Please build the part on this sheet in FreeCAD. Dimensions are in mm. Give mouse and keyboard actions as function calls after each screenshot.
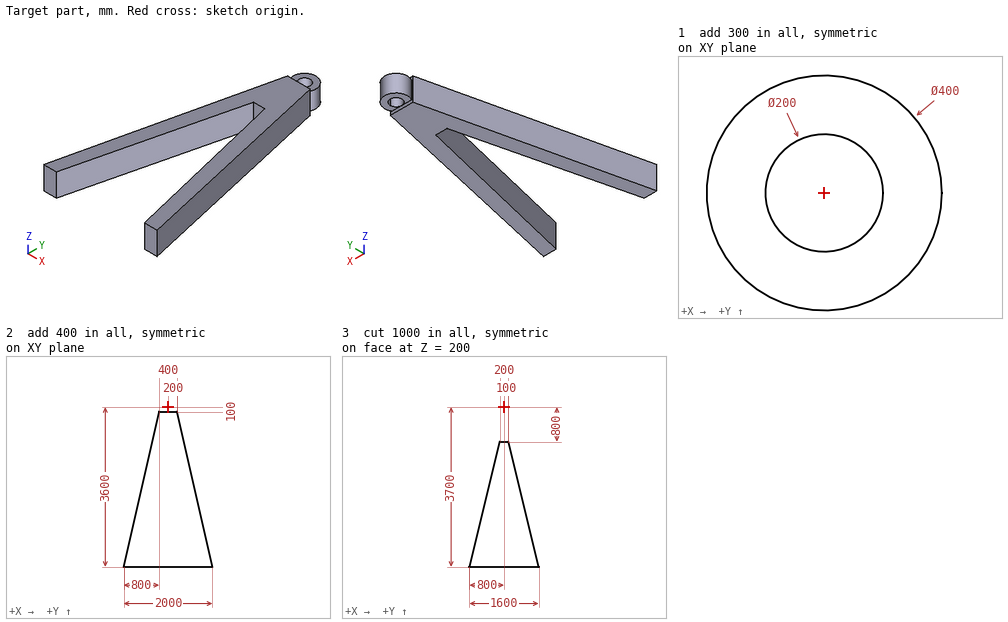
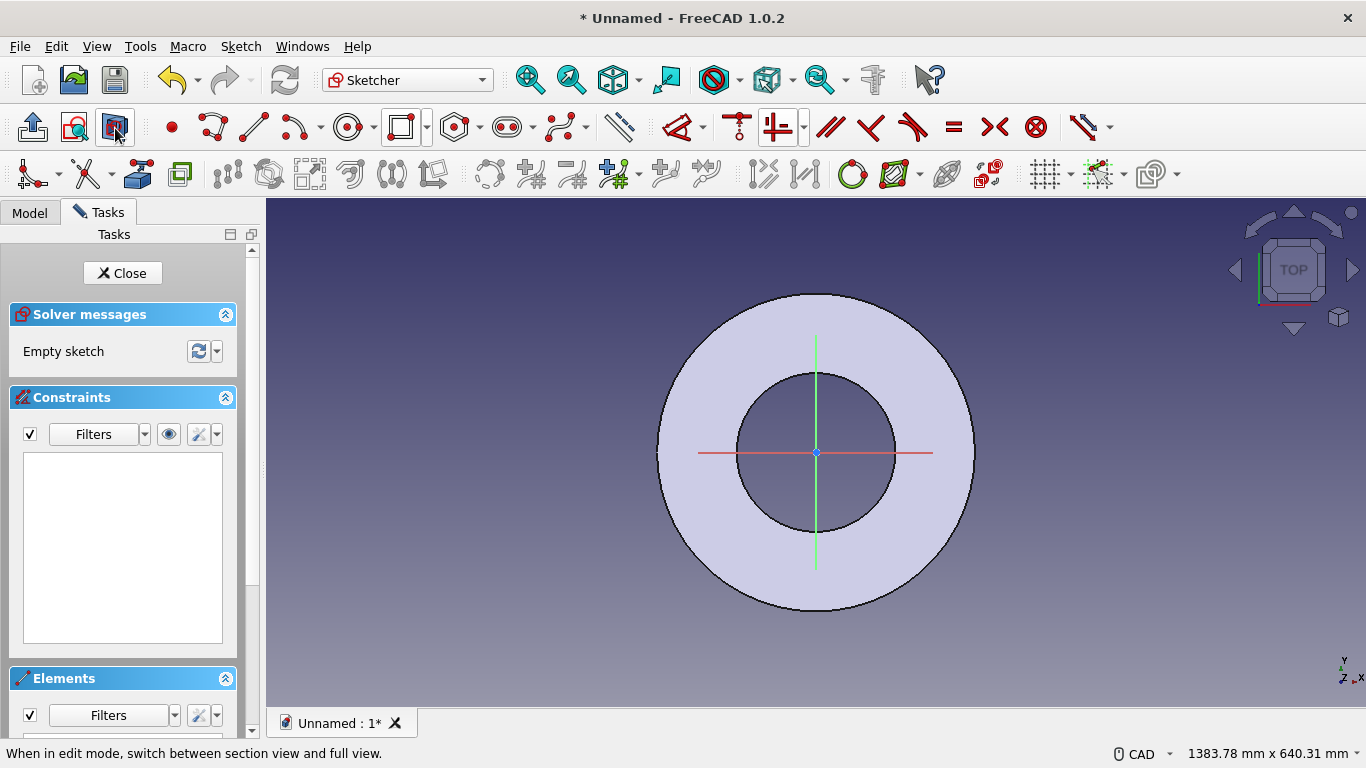
scroll(739, 274, down, 11)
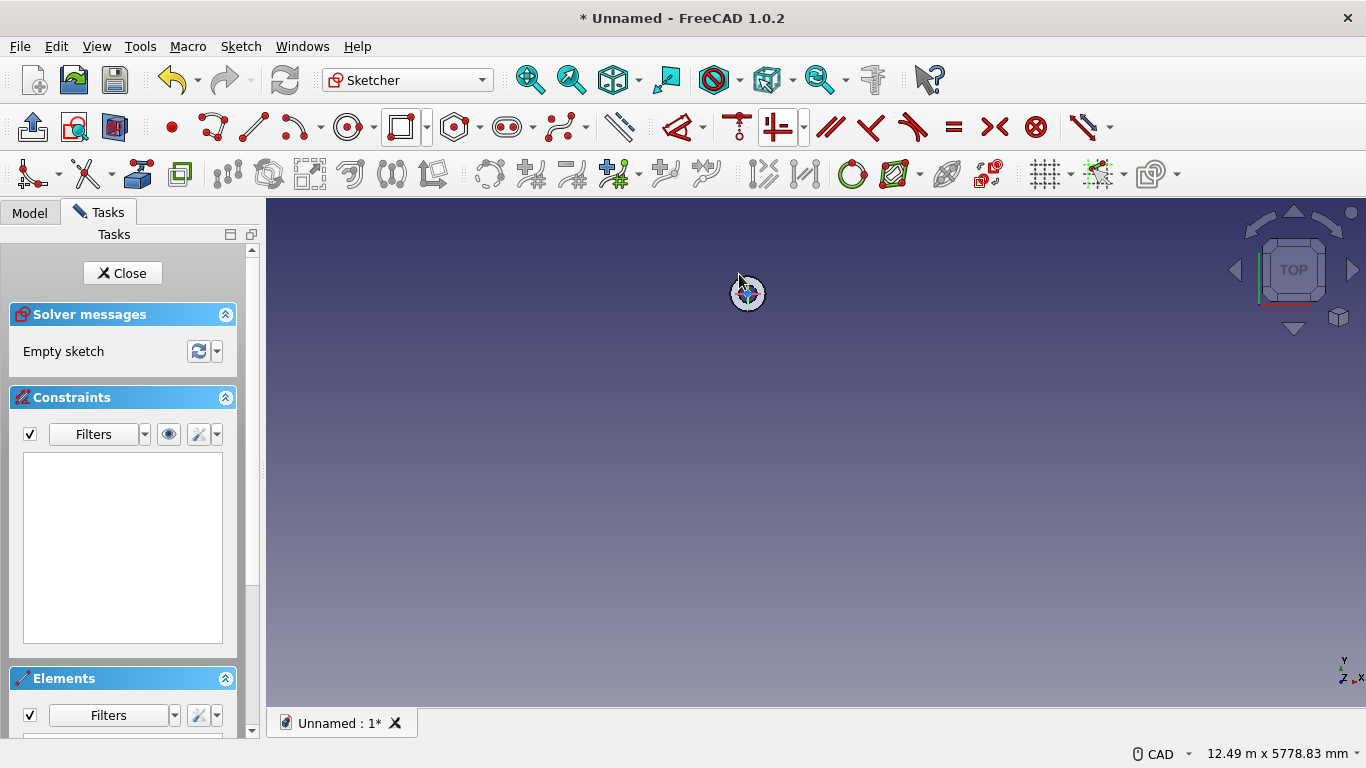
click(213, 128)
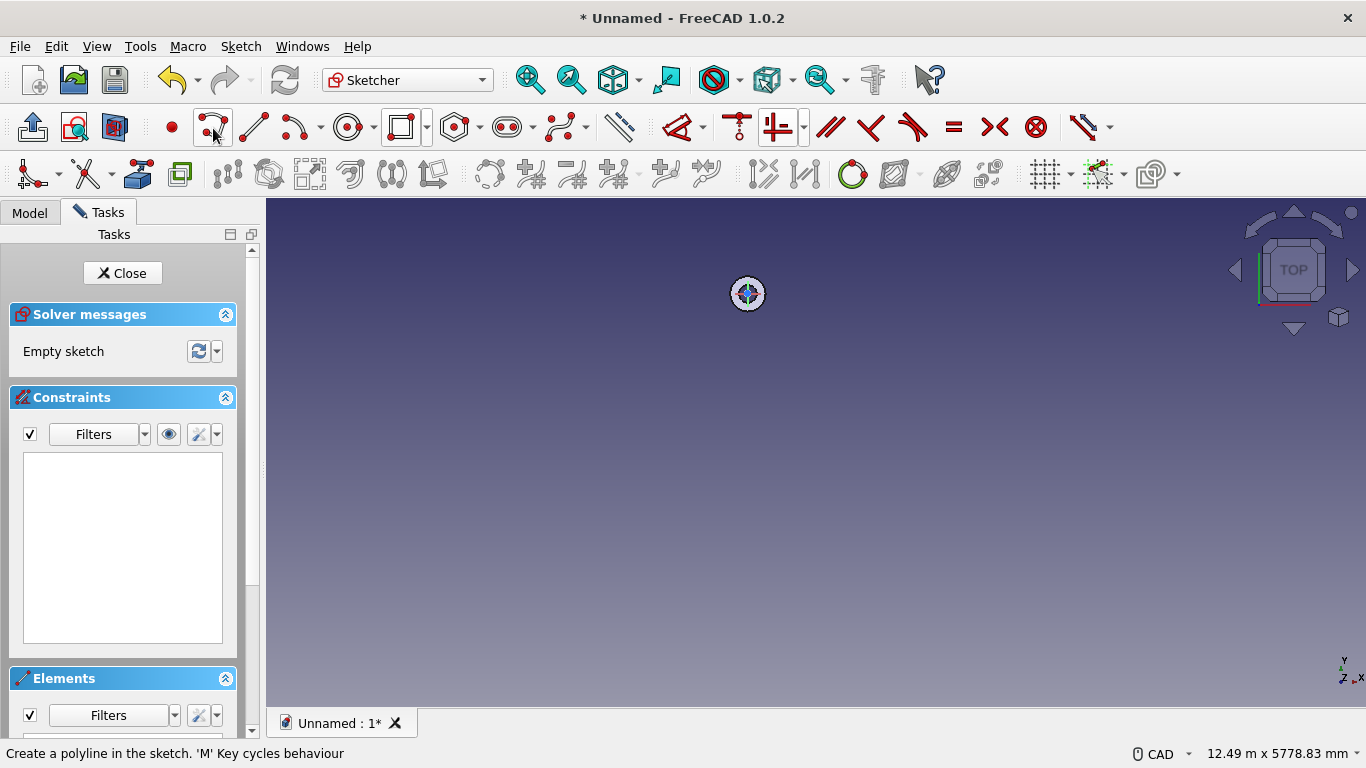
scroll(766, 303, up, 3)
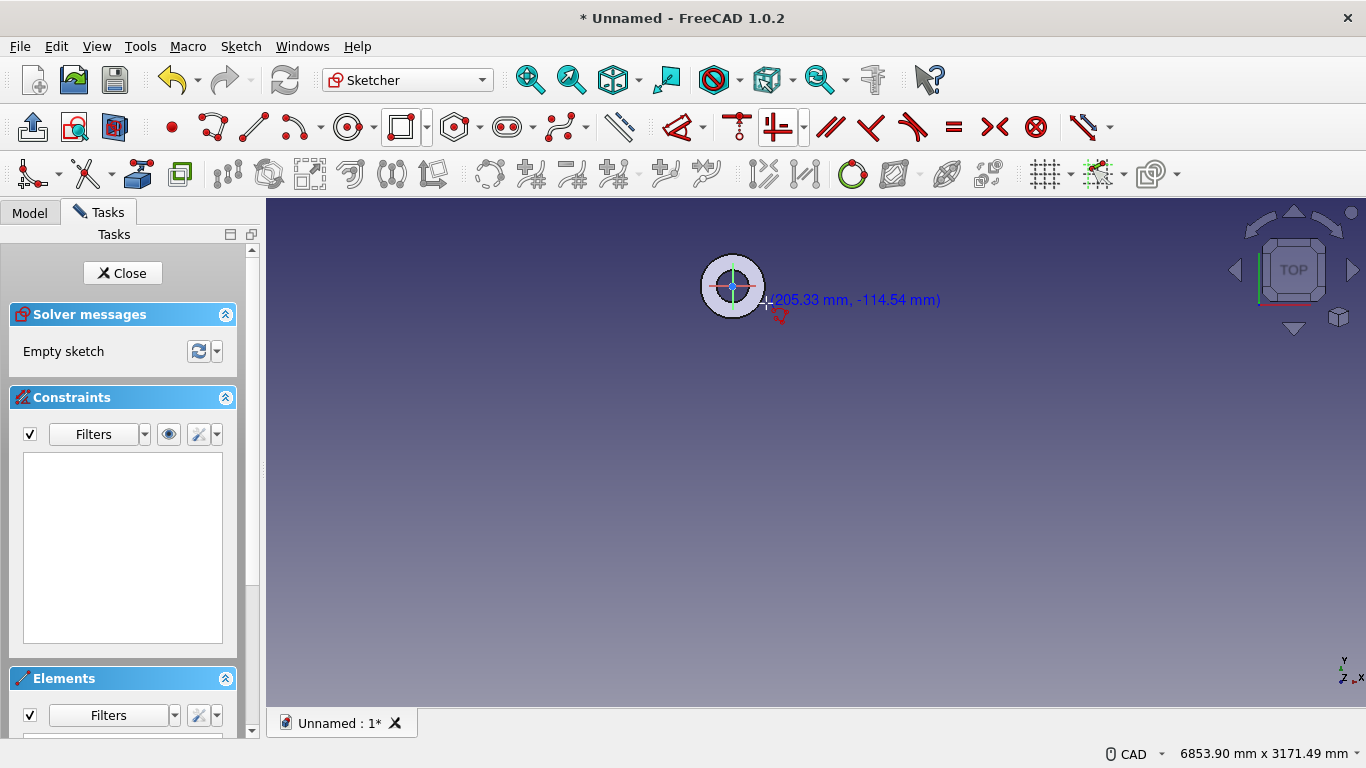
click(765, 302)
click(701, 302)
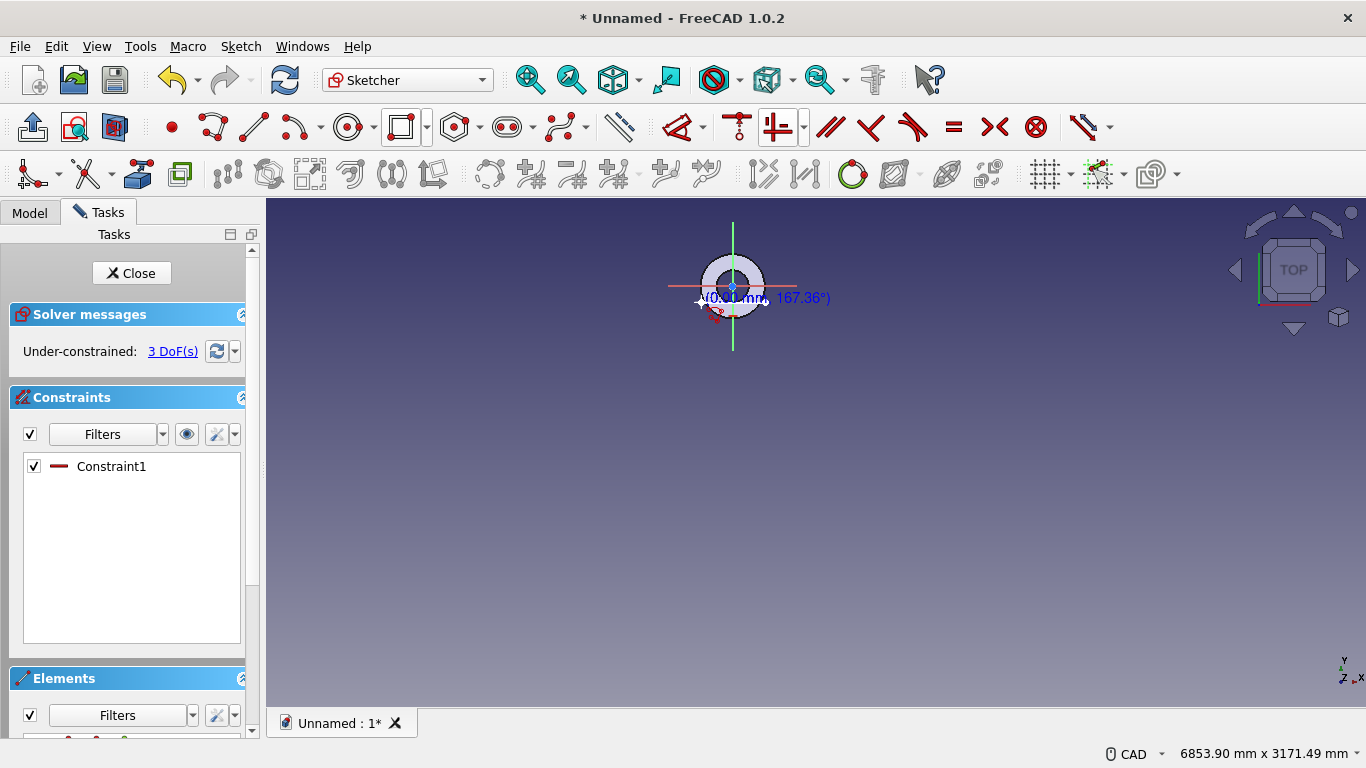
scroll(766, 303, down, 3)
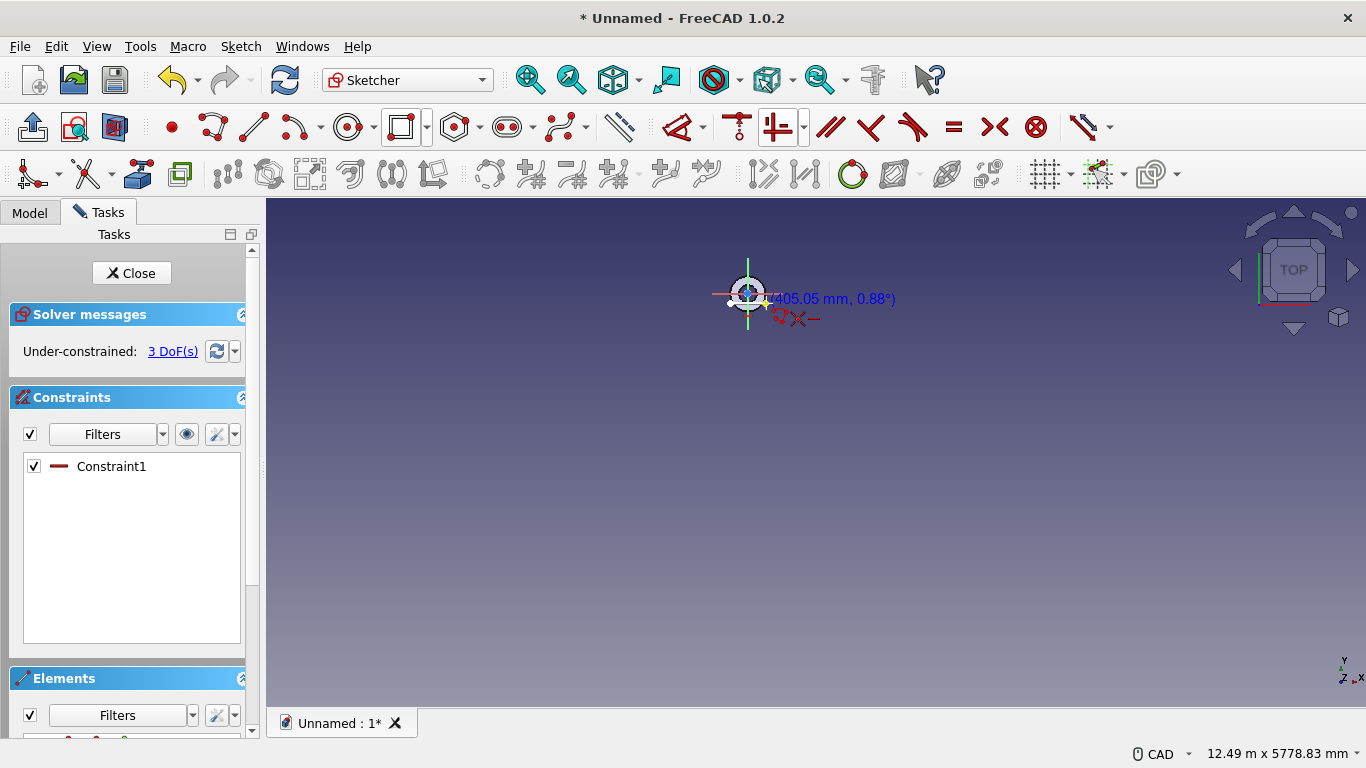
click(660, 611)
click(836, 611)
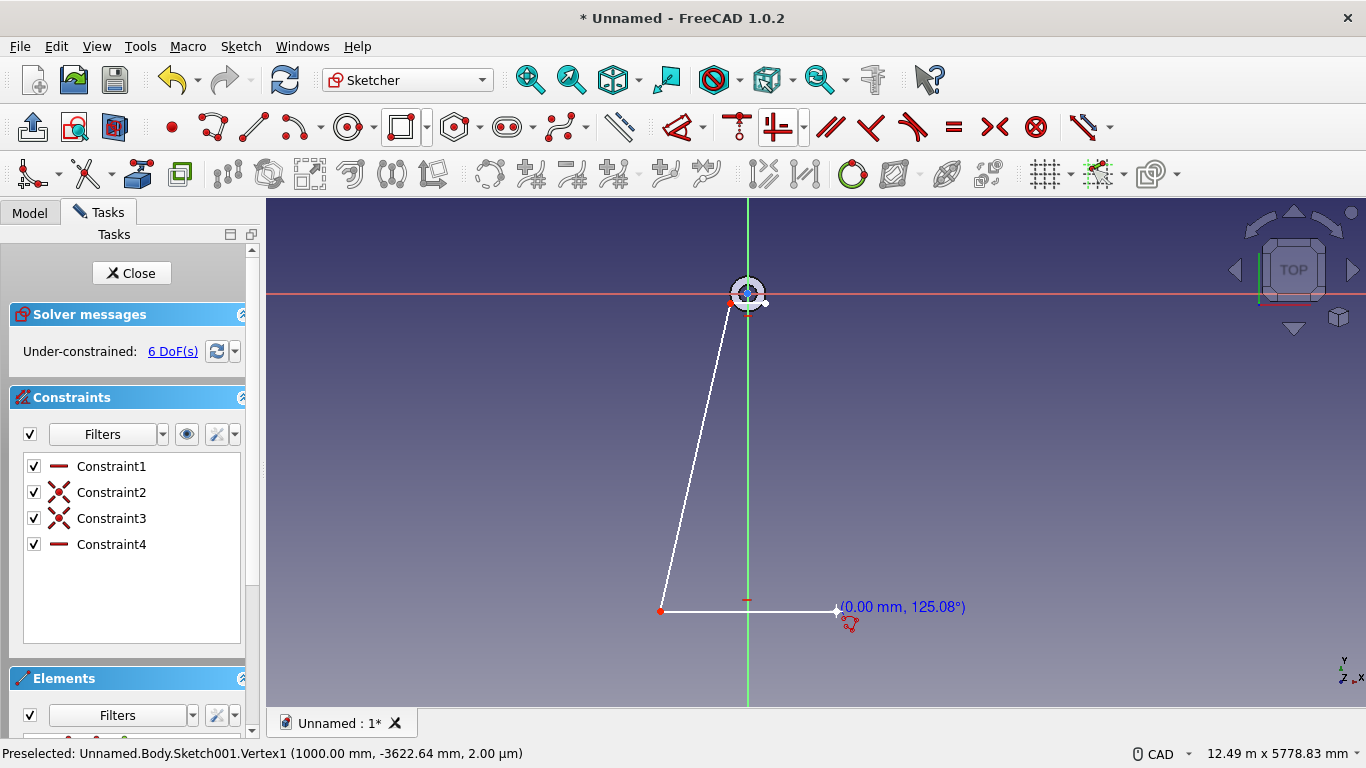
scroll(766, 303, up, 3)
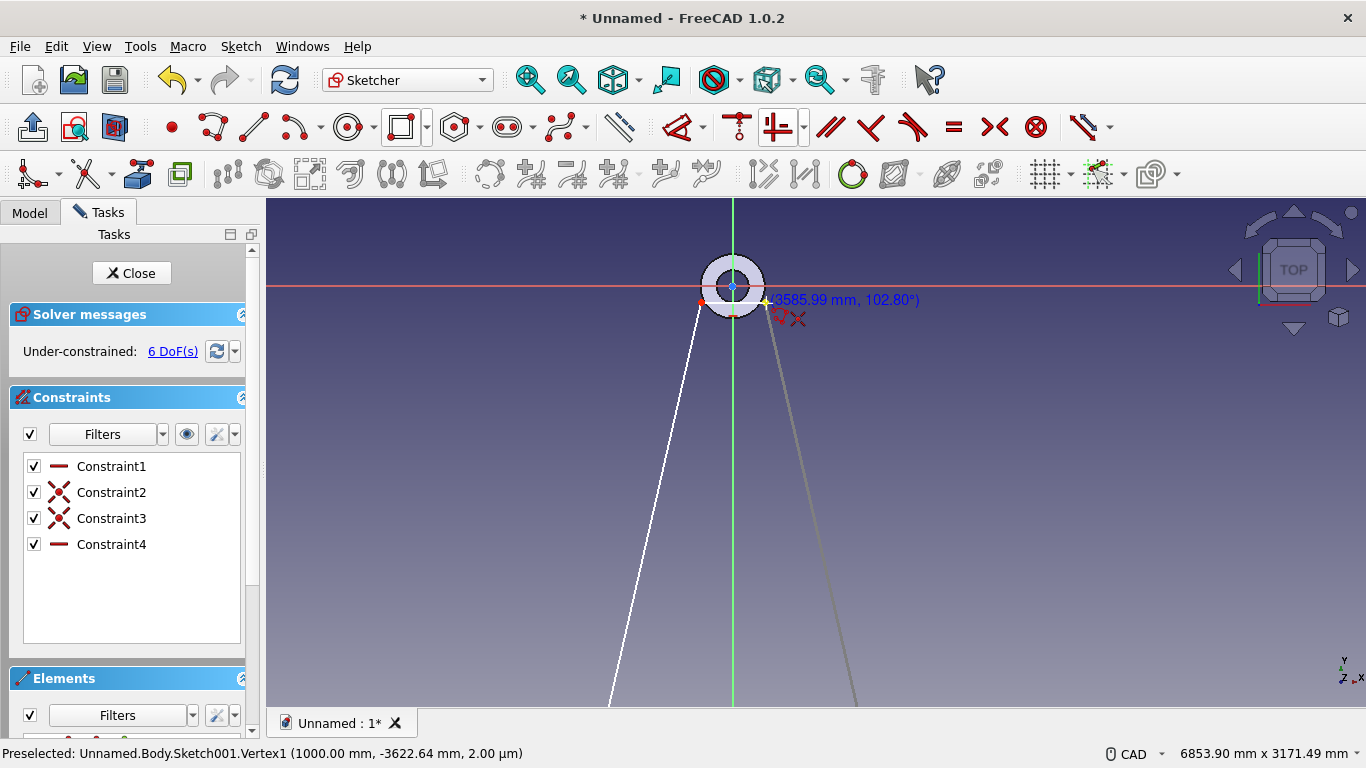
click(765, 303)
key(Escape)
key(Escape)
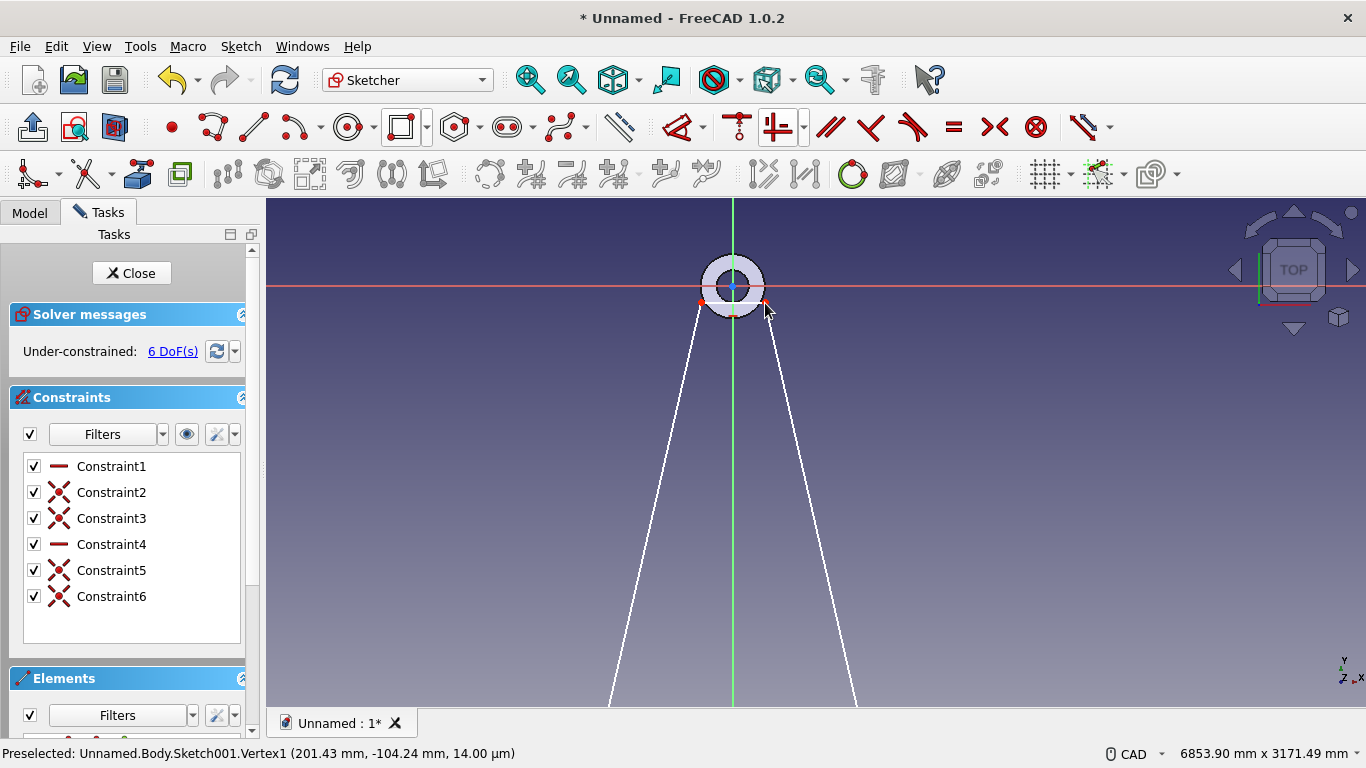
click(676, 128)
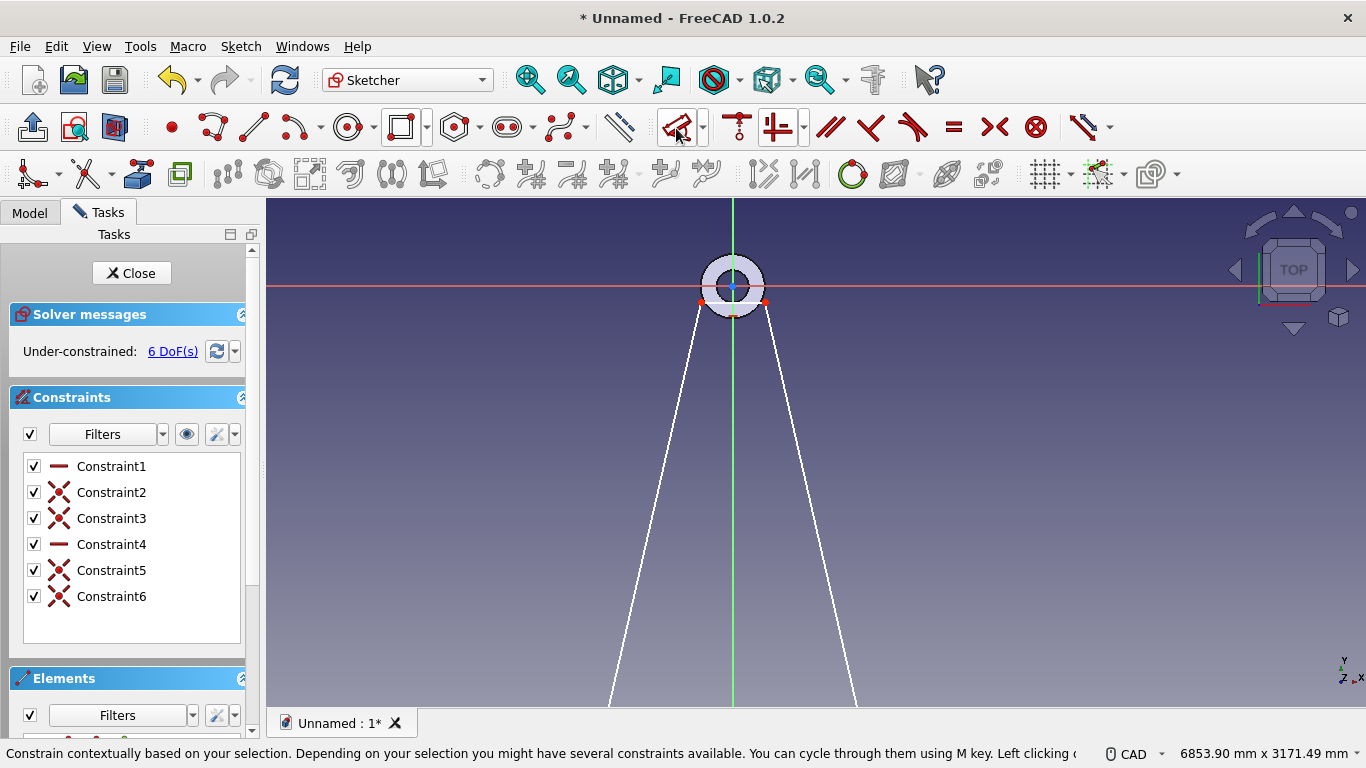
click(746, 303)
click(718, 269)